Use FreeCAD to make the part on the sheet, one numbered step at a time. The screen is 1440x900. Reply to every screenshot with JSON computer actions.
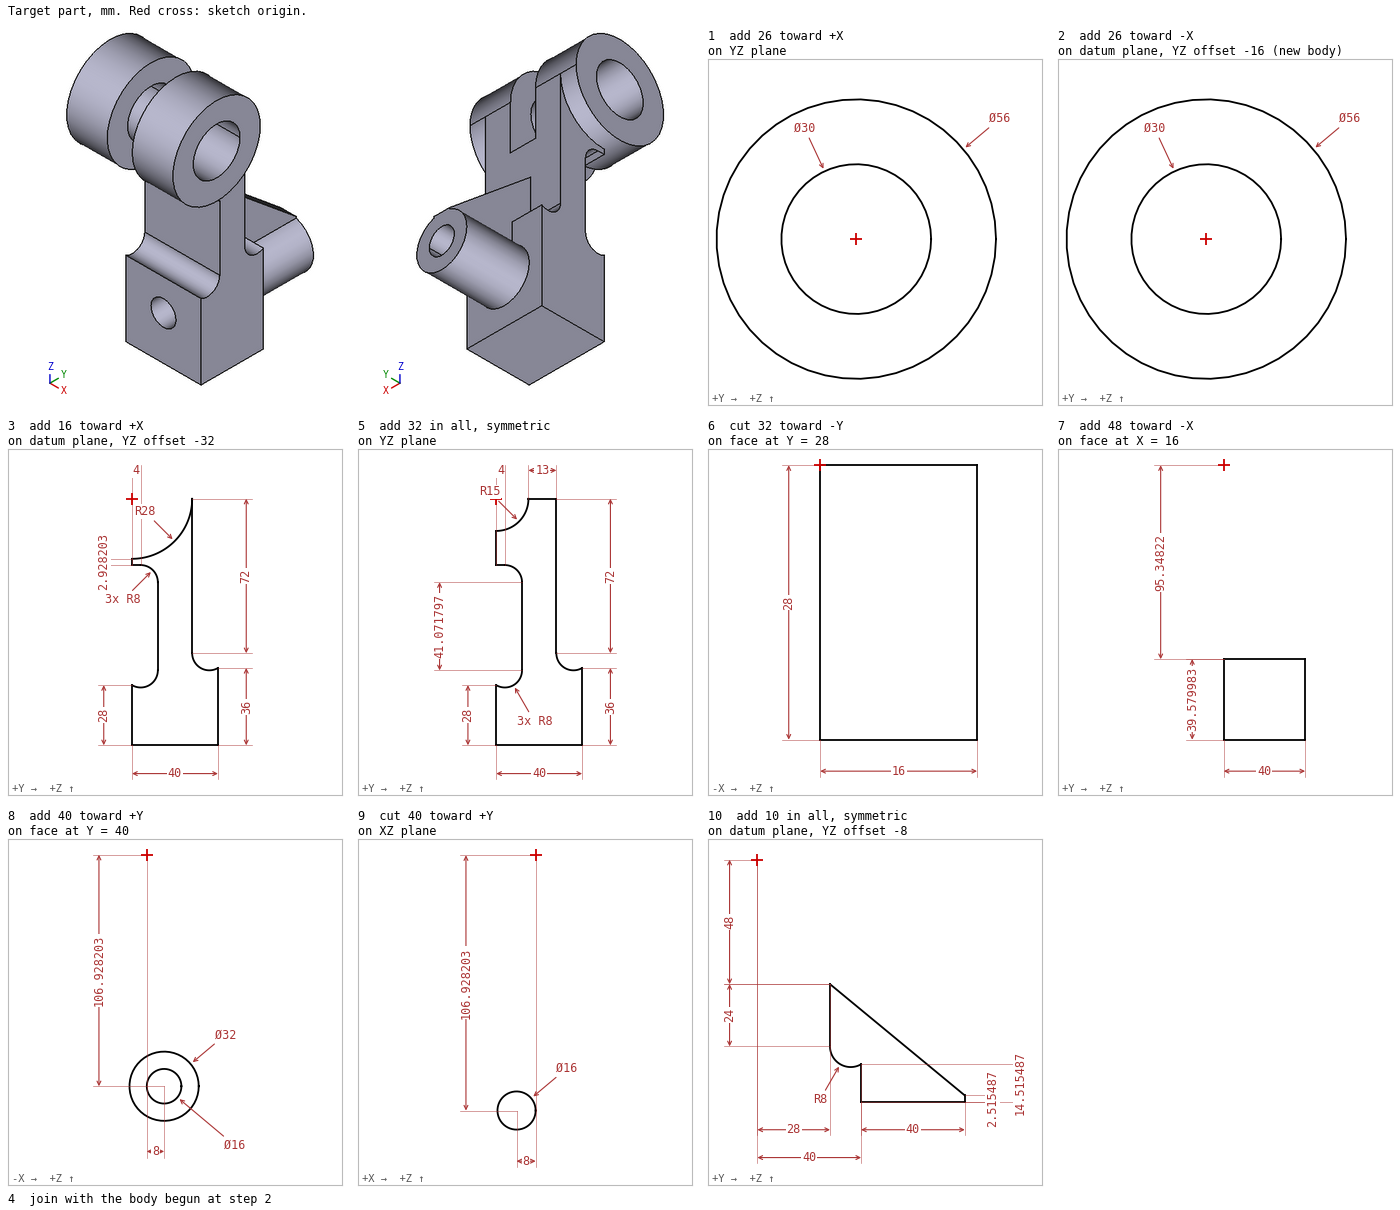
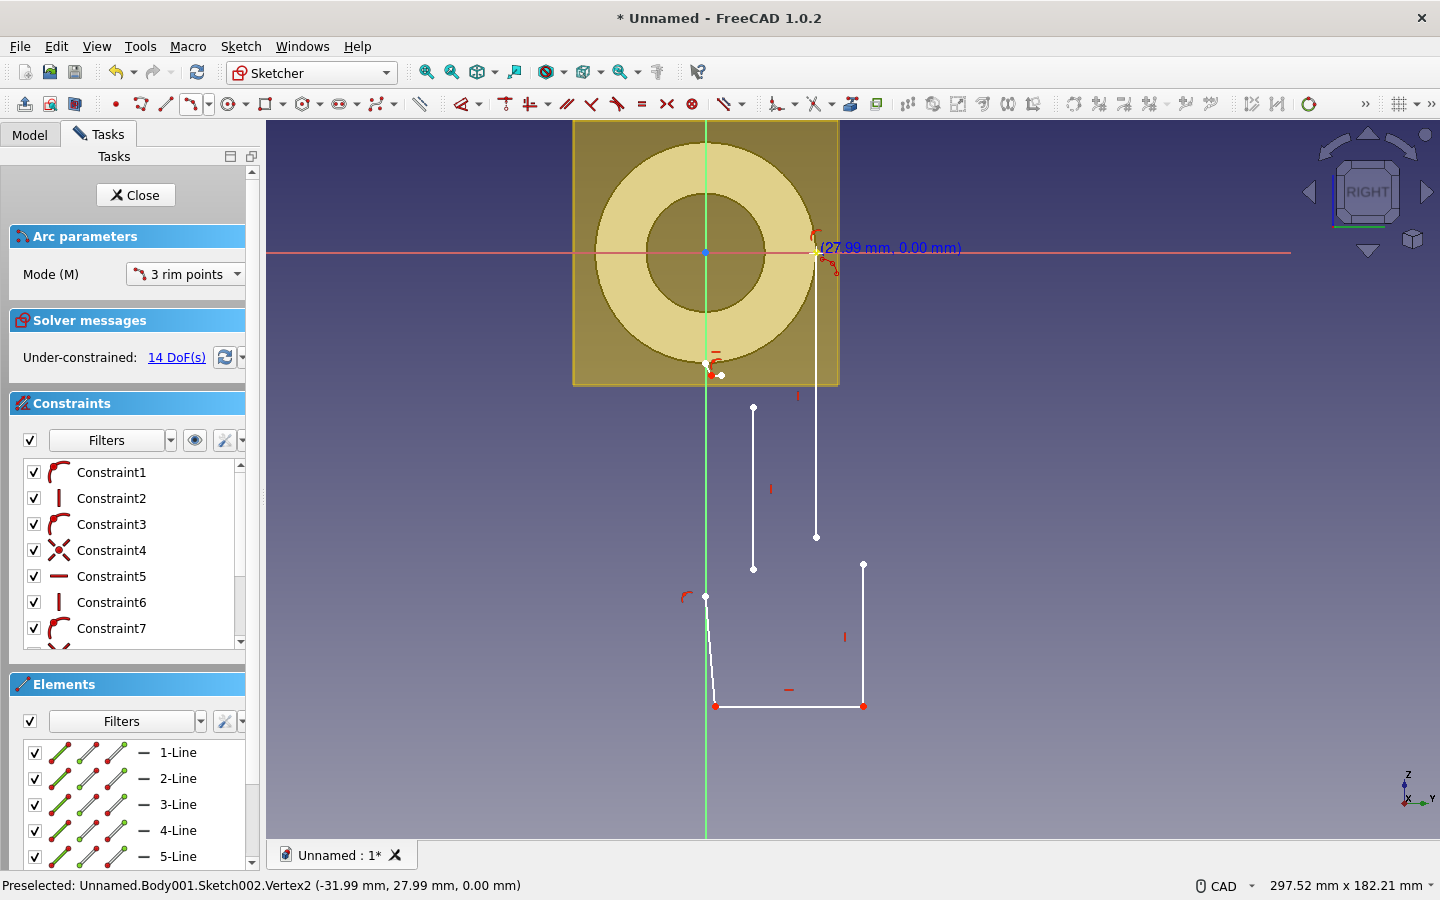
{"action": "scroll", "coordinate": [706, 363], "scroll_direction": "up", "scroll_amount": 6}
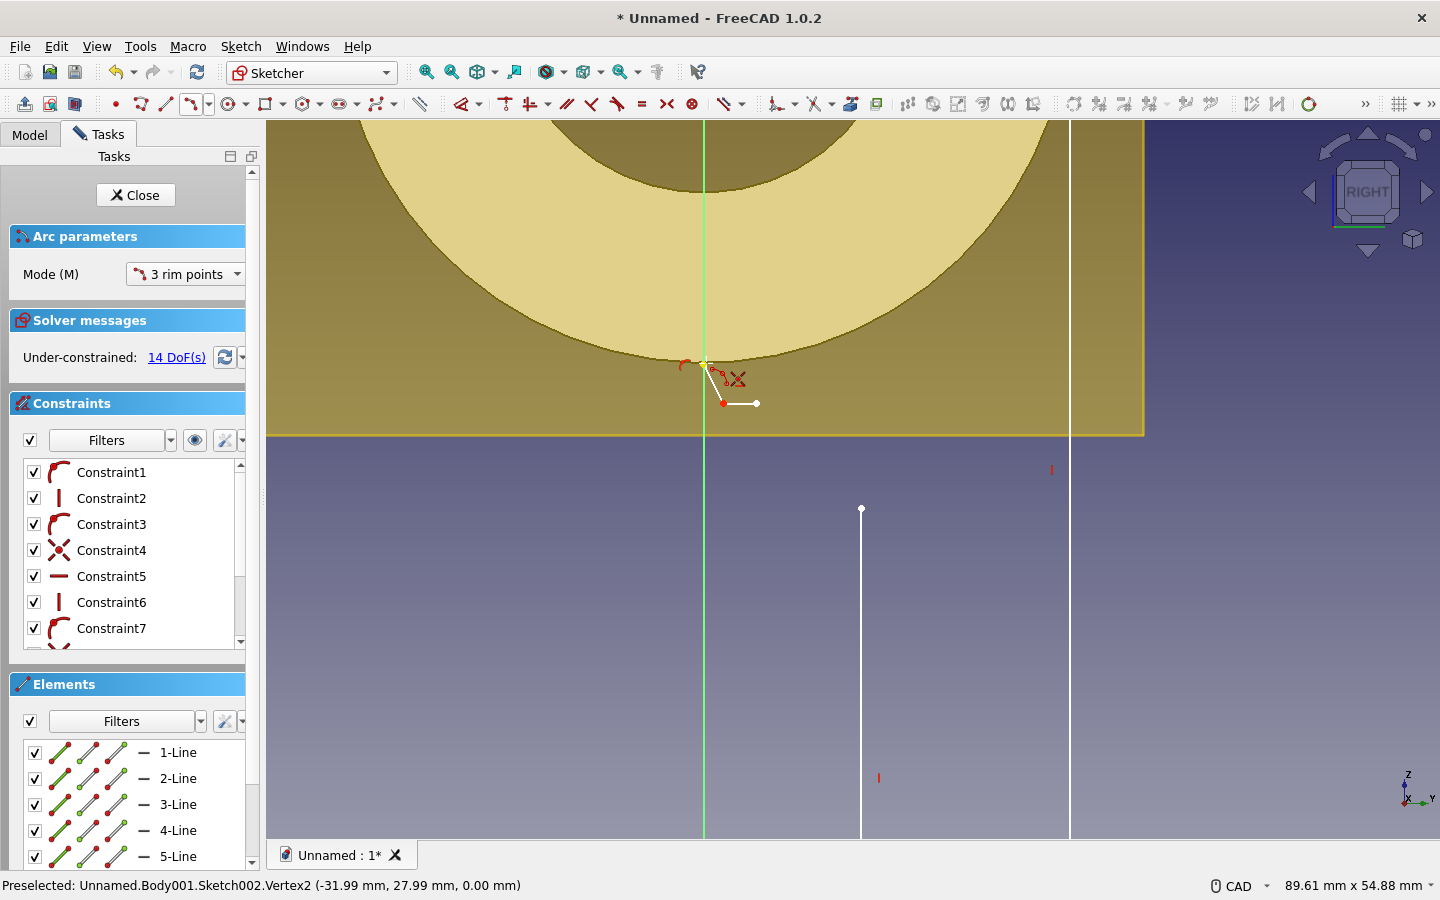
{"action": "left_click", "coordinate": [704, 365]}
{"action": "left_click", "coordinate": [963, 255]}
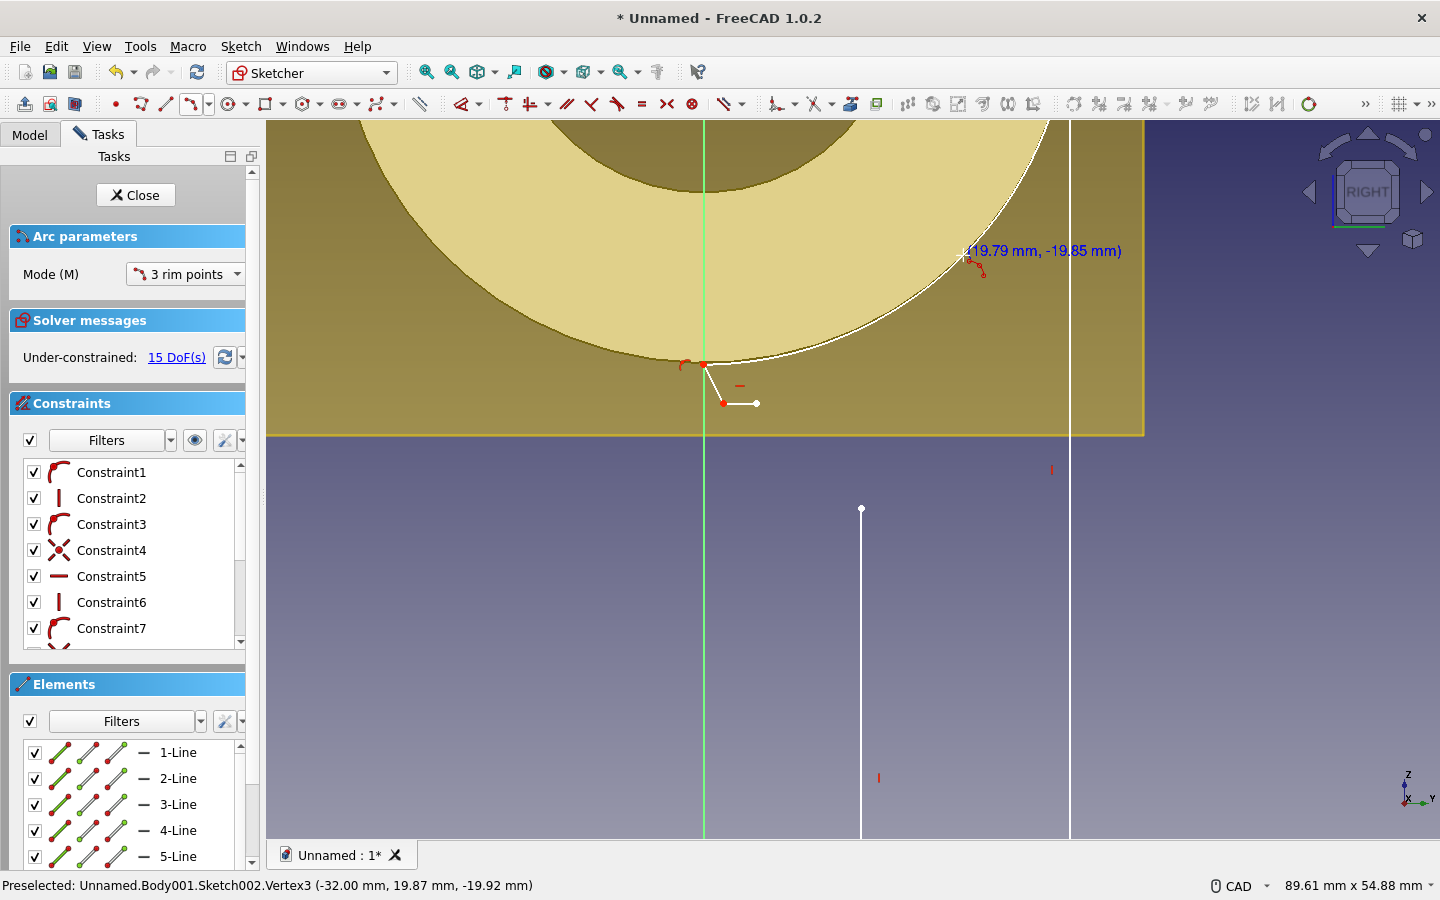
{"action": "left_click", "coordinate": [757, 404]}
{"action": "left_click", "coordinate": [861, 509]}
{"action": "left_click", "coordinate": [830, 432]}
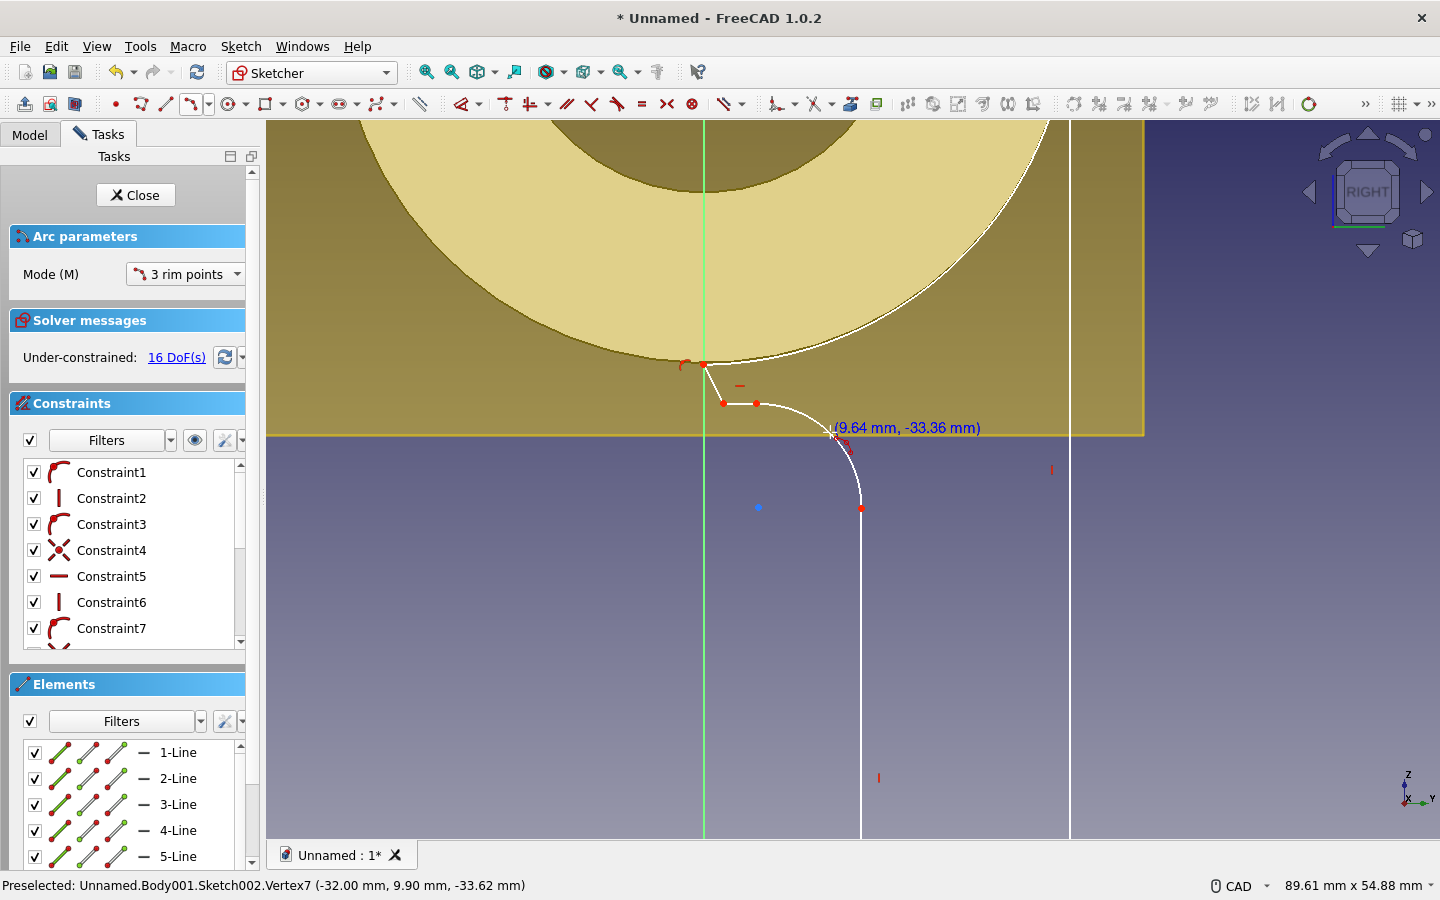
{"action": "scroll", "coordinate": [706, 363], "scroll_direction": "down", "scroll_amount": 6}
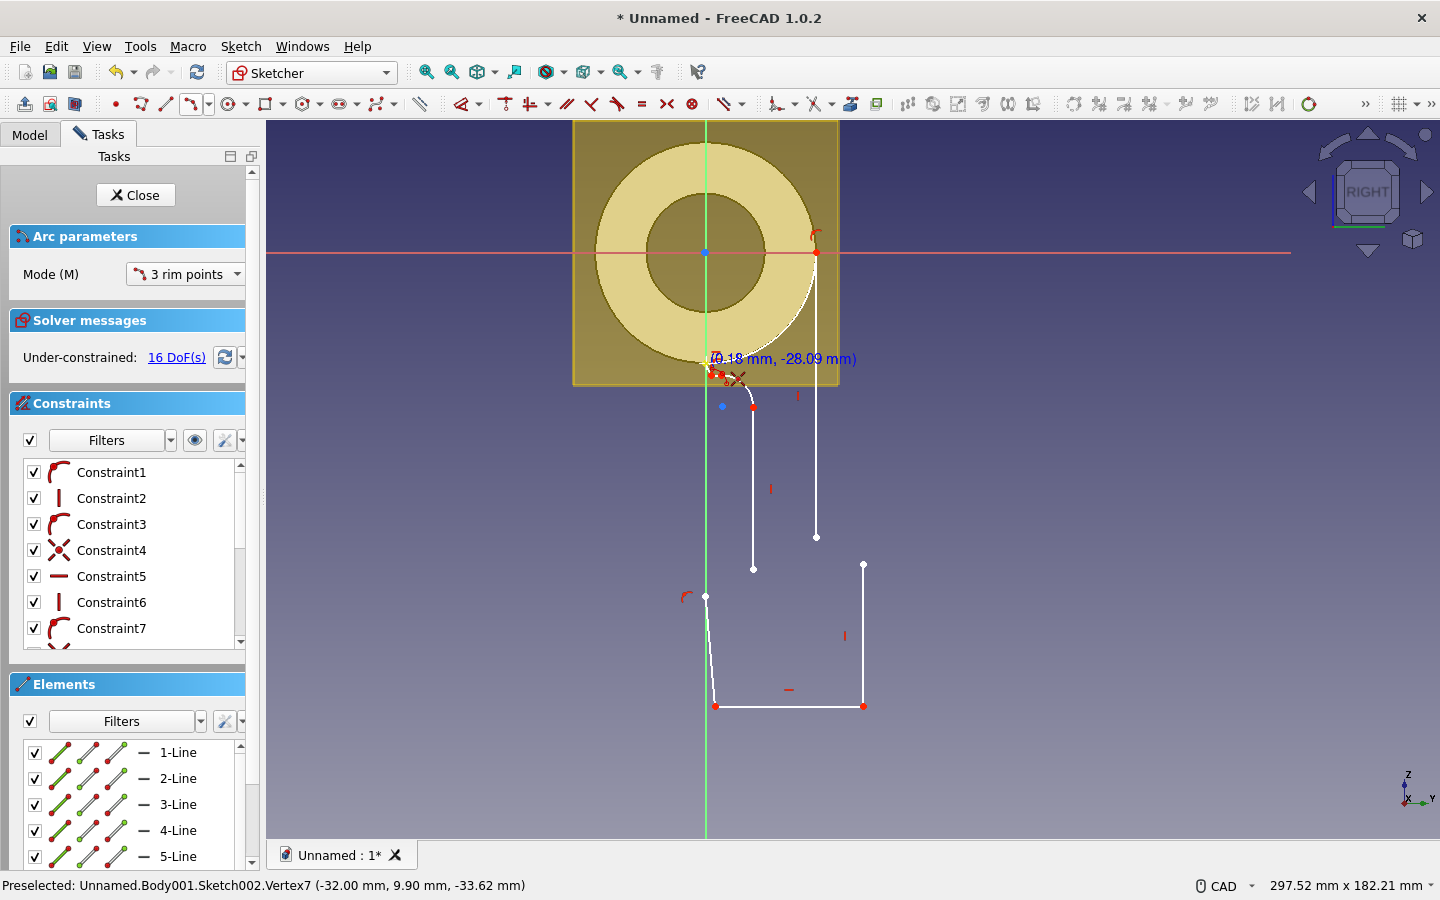
{"action": "left_click", "coordinate": [753, 569]}
{"action": "left_click", "coordinate": [706, 596]}
{"action": "left_click", "coordinate": [737, 596]}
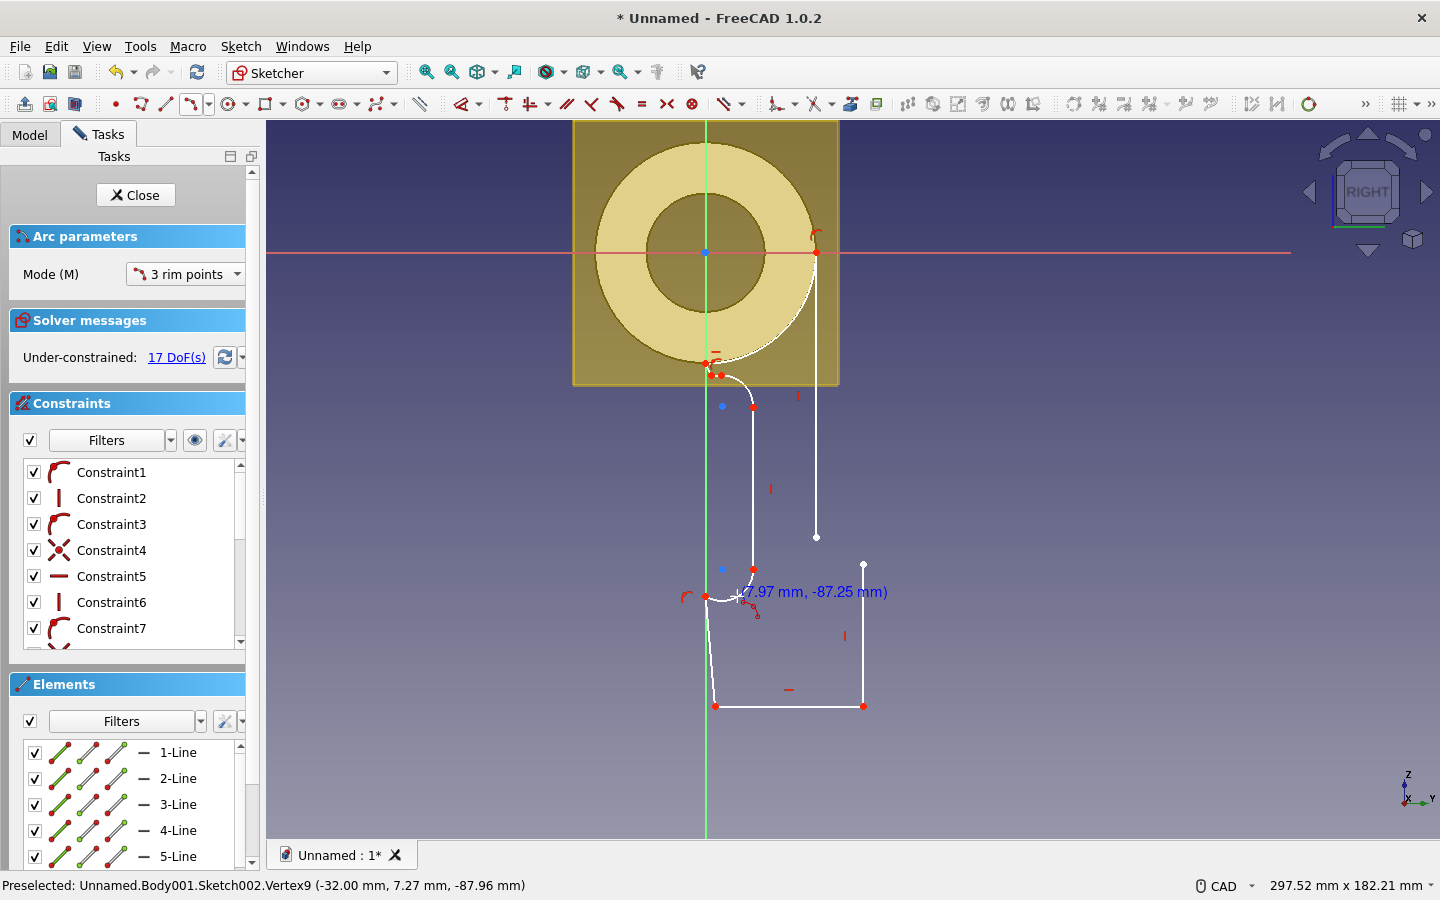
{"action": "left_click", "coordinate": [863, 565]}
{"action": "left_click", "coordinate": [816, 538]}
{"action": "left_click", "coordinate": [832, 564]}
{"action": "key", "text": "Escape"}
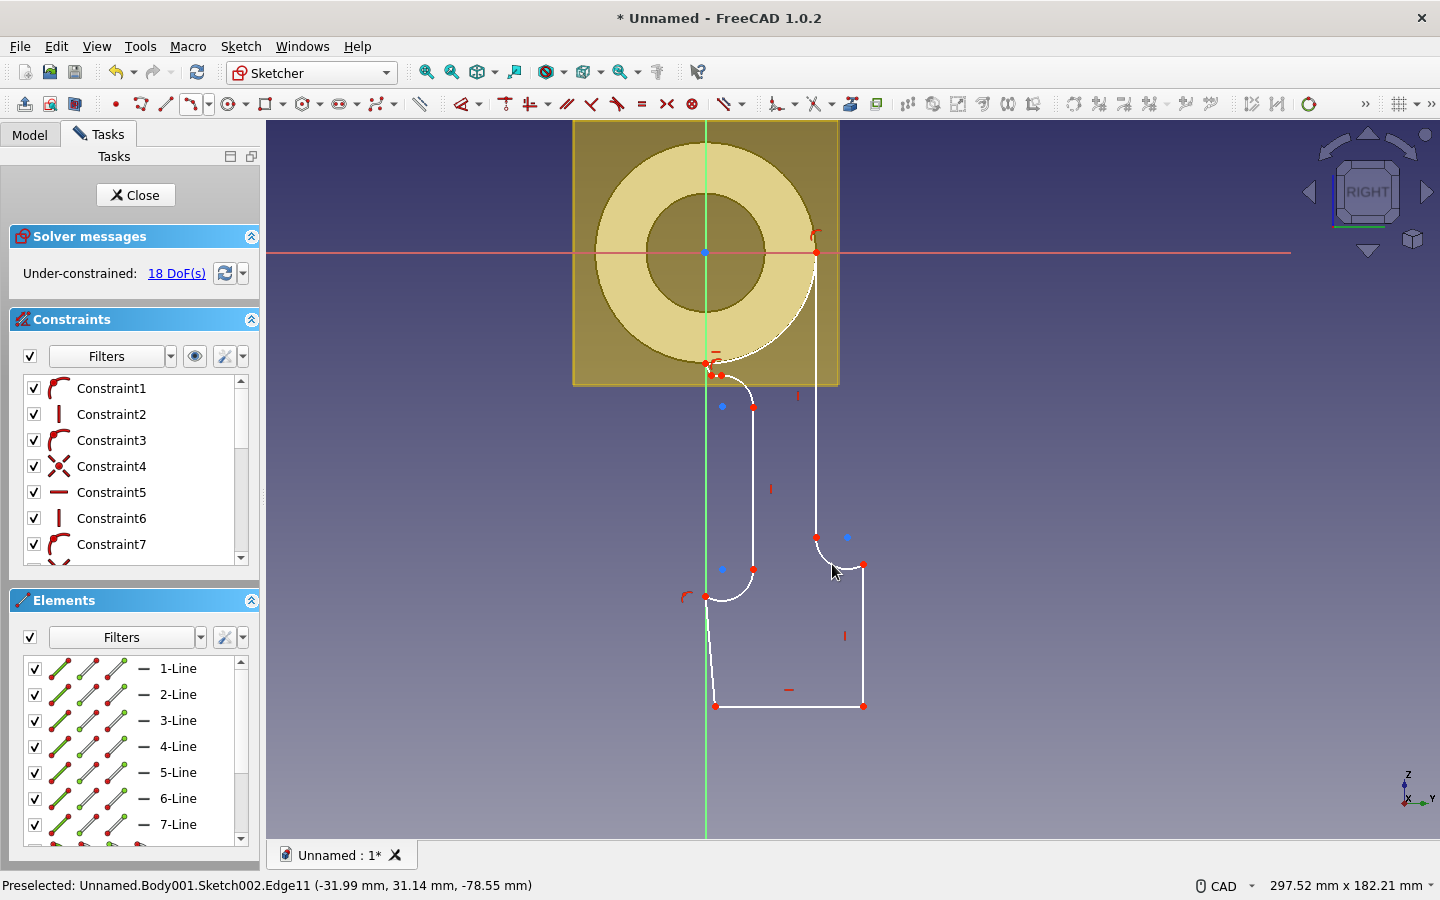
{"action": "left_click", "coordinate": [816, 452]}